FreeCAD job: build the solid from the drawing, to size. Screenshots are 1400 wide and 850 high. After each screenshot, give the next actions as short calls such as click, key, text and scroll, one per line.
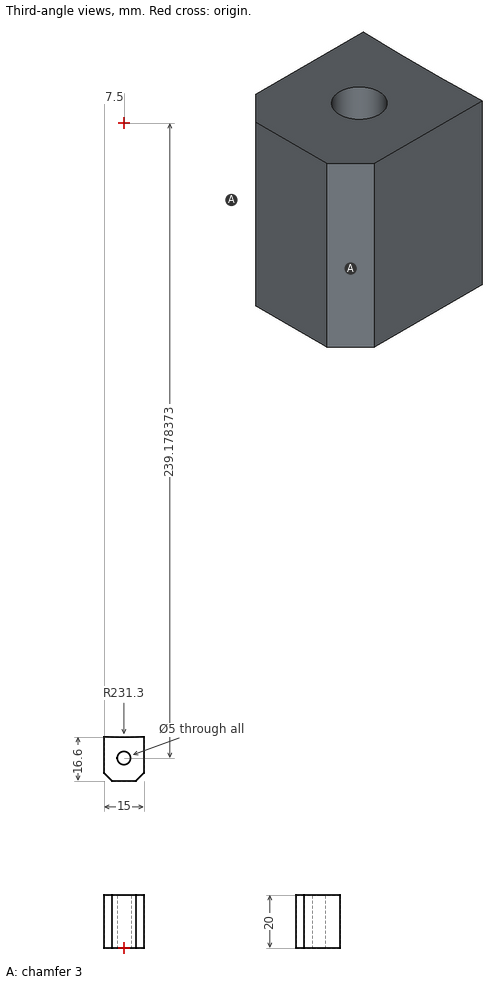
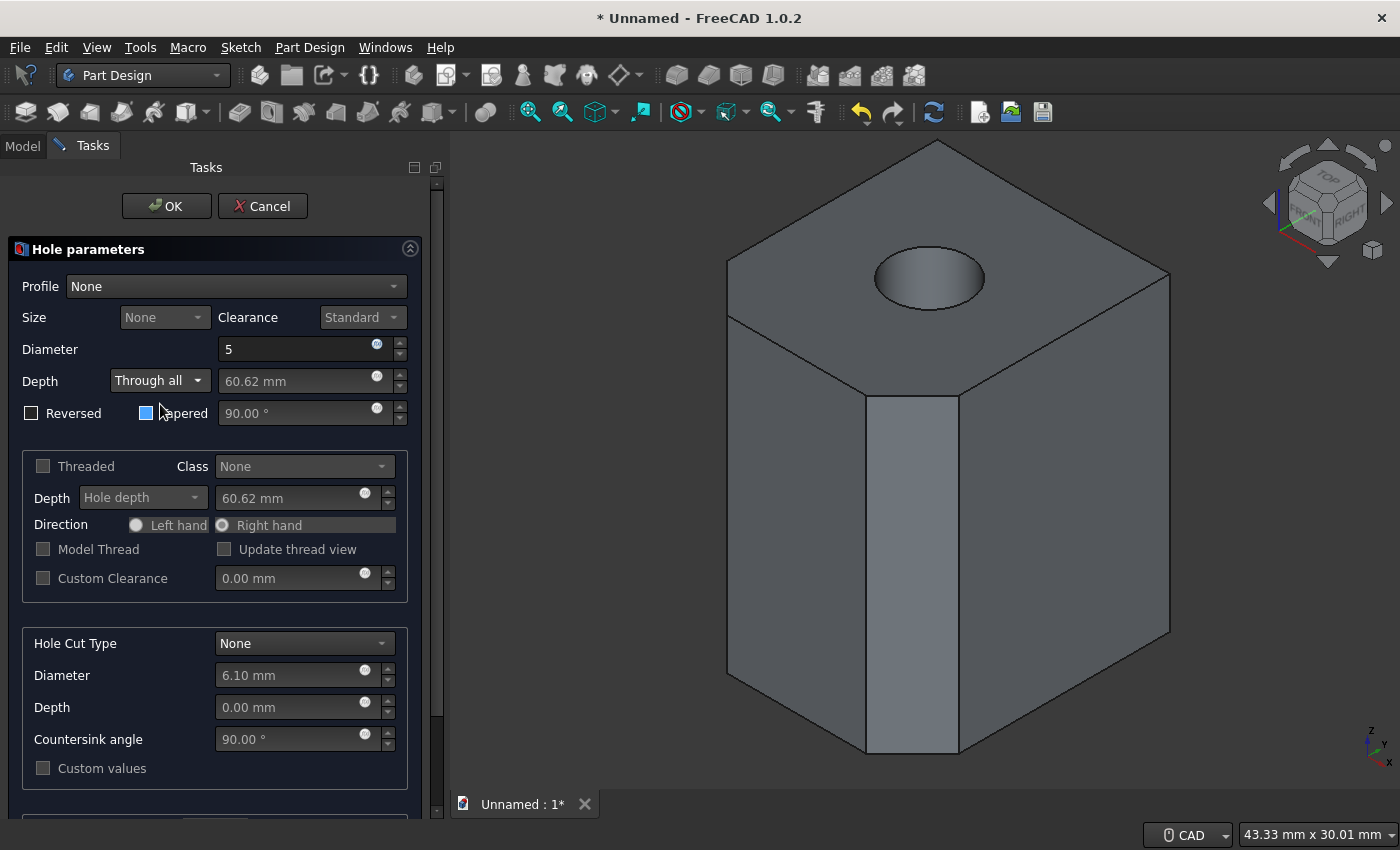
click(167, 206)